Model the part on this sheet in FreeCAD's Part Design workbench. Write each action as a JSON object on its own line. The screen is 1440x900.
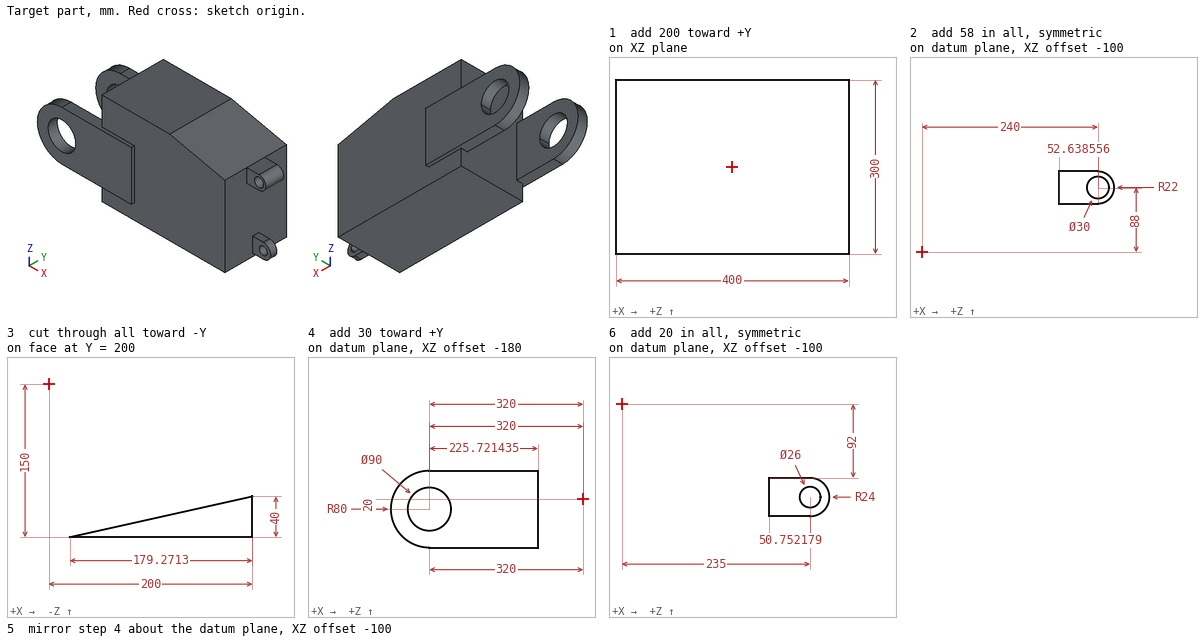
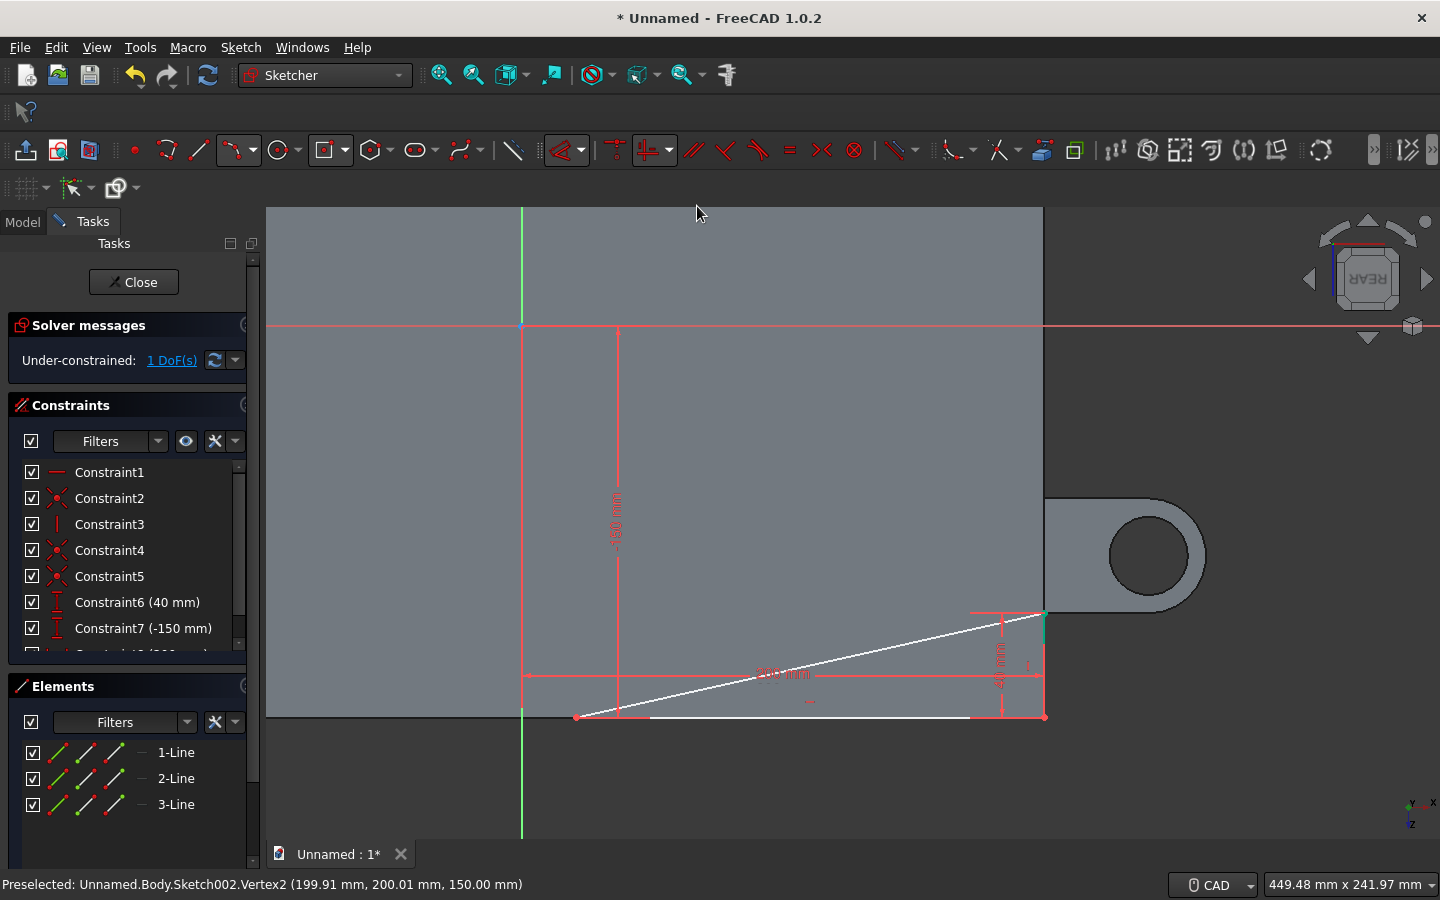
{"action": "left_click", "coordinate": [716, 718]}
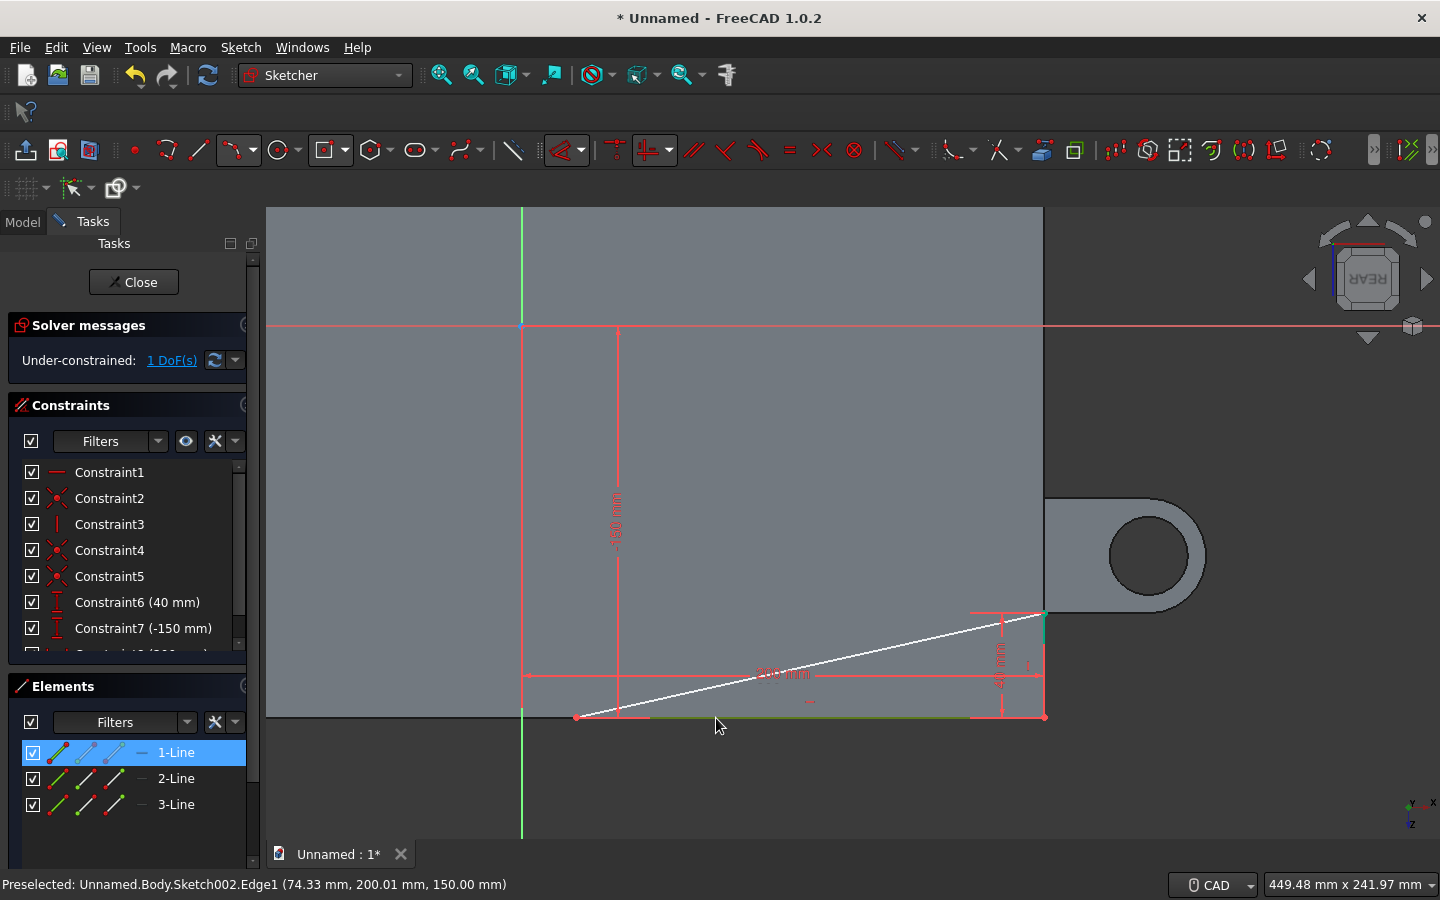
{"action": "key", "text": "l"}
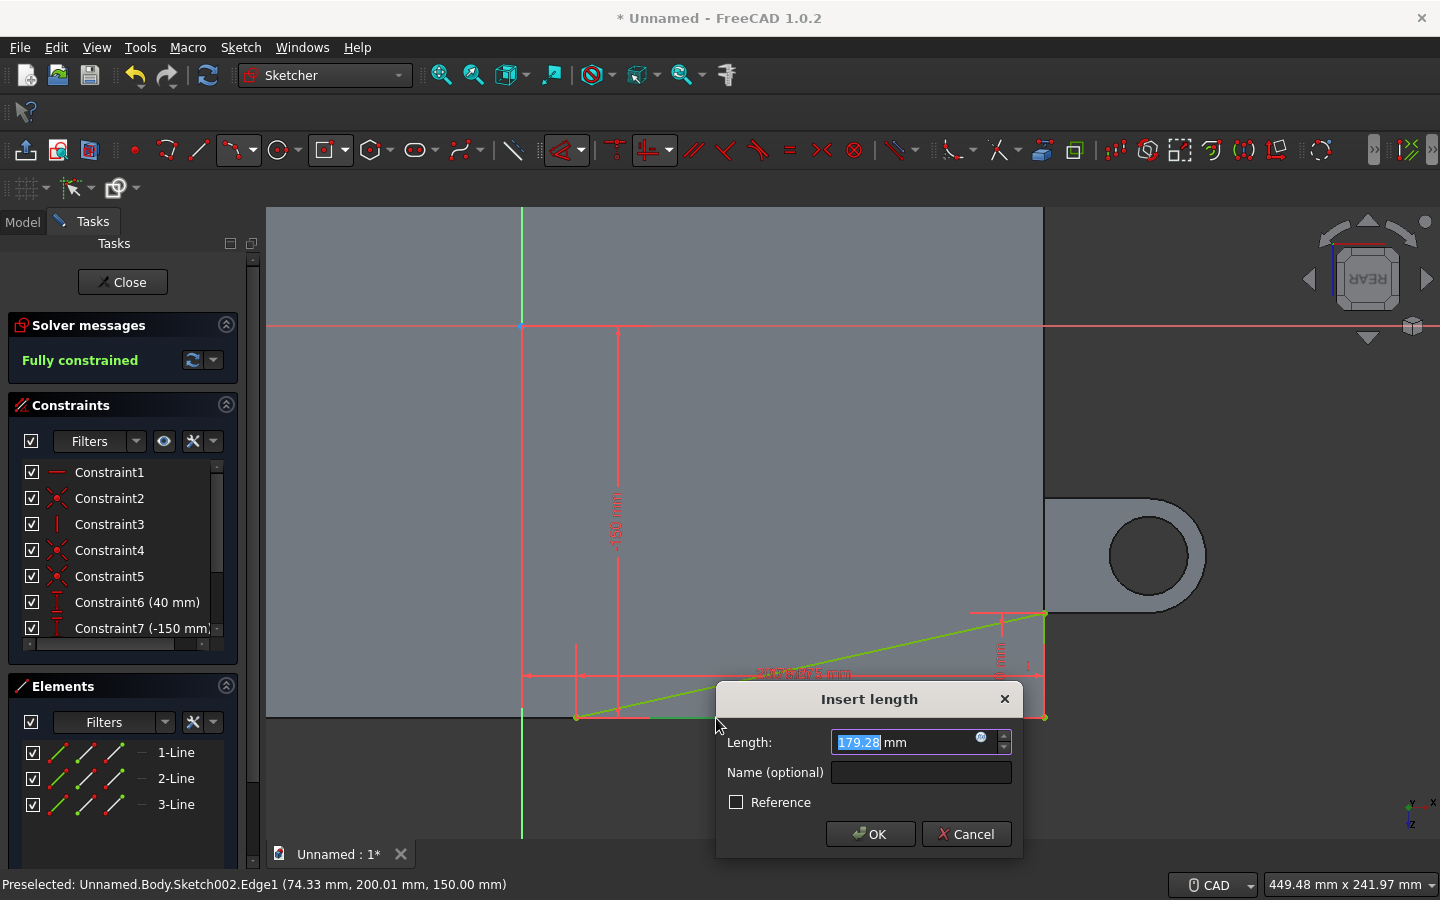
{"action": "type", "text": "179.2713"}
{"action": "key", "text": "Return"}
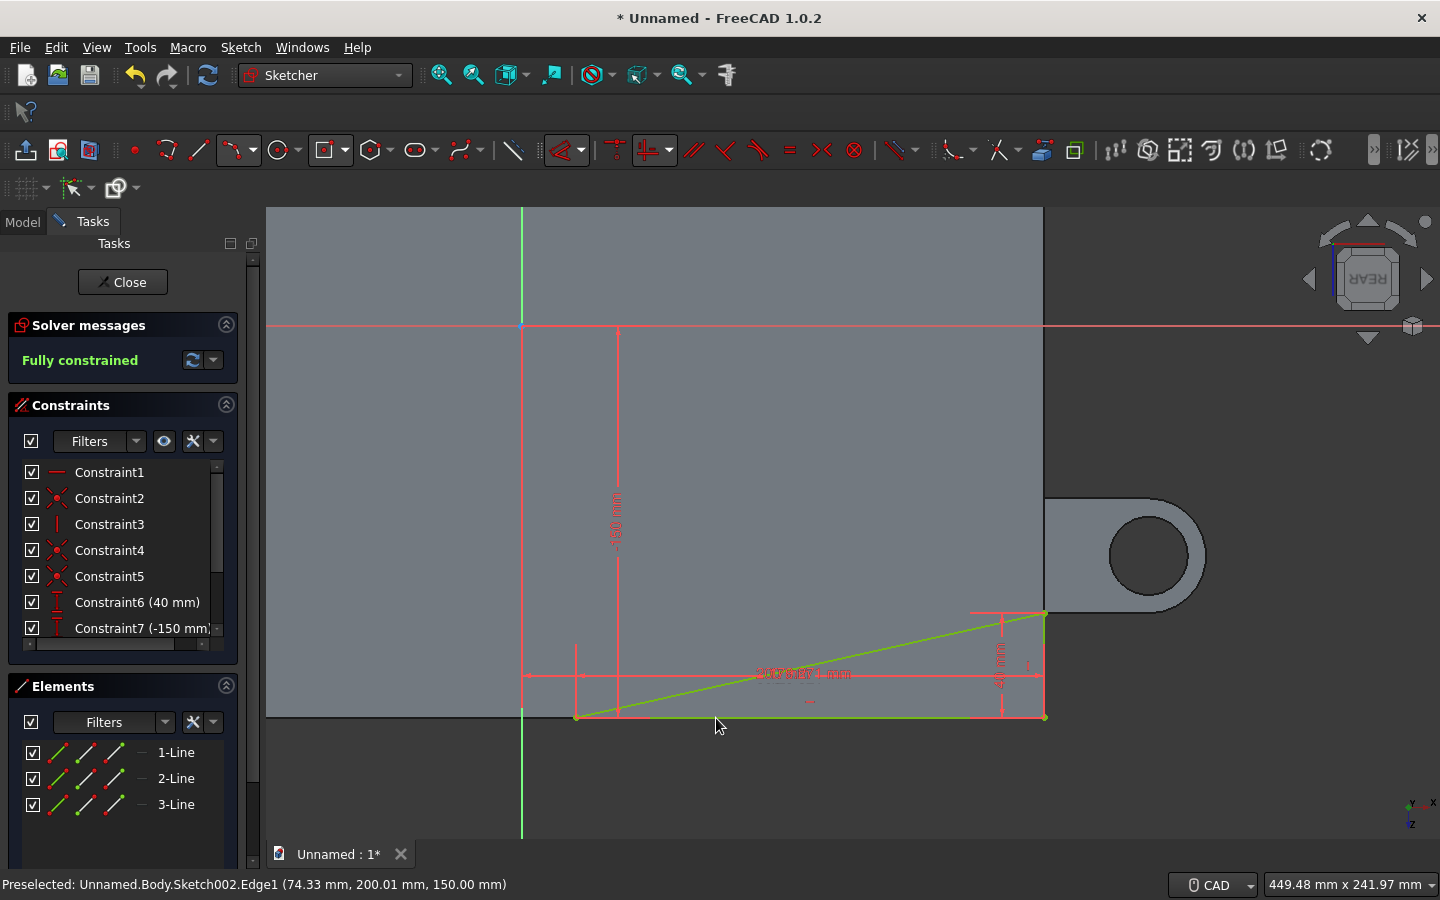
{"action": "left_click", "coordinate": [123, 282]}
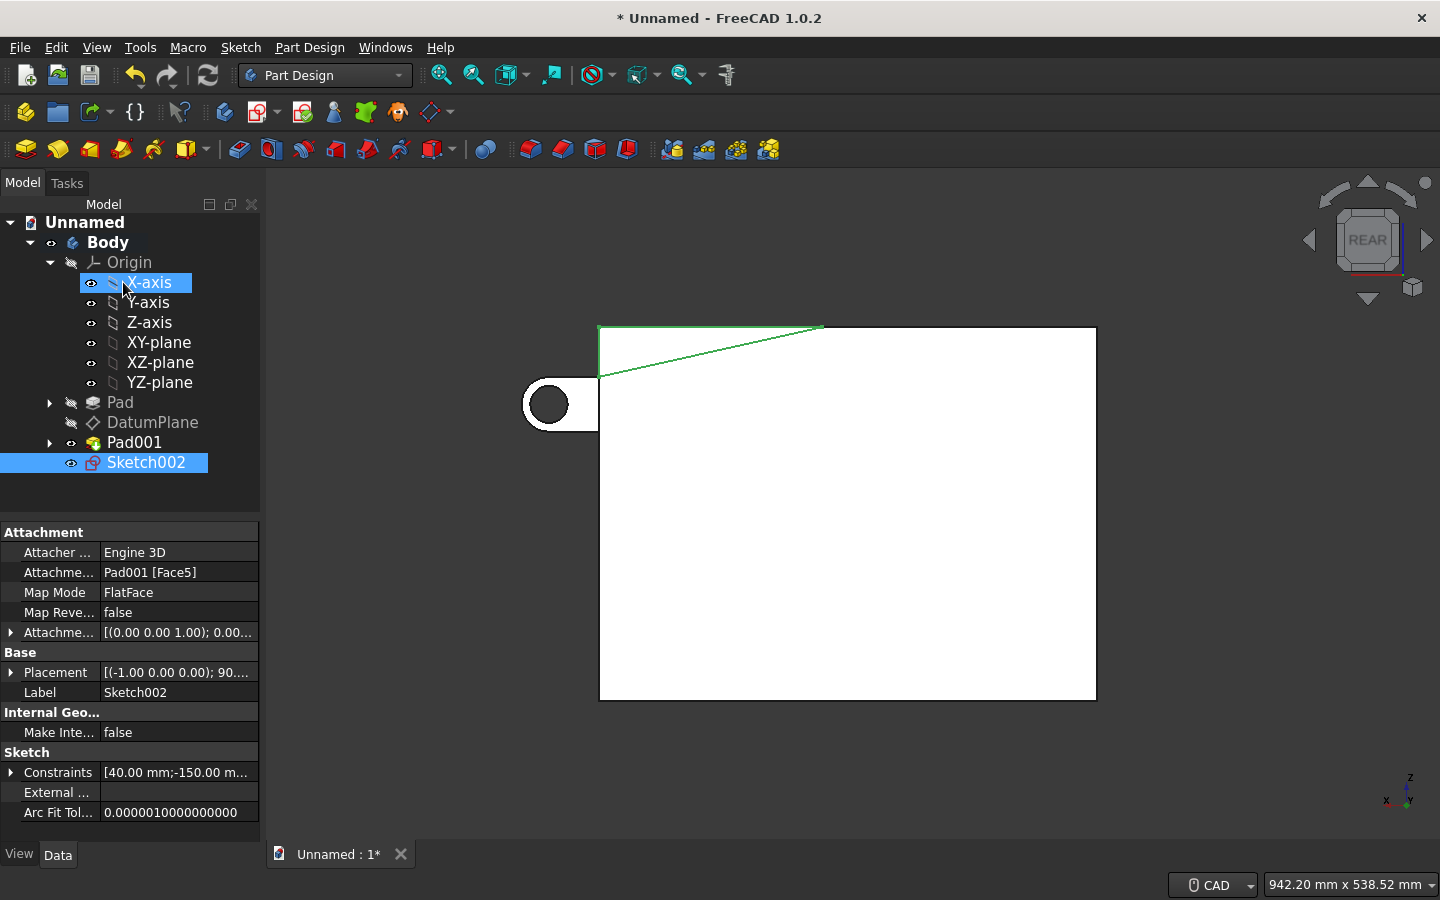
{"action": "left_click", "coordinate": [240, 150]}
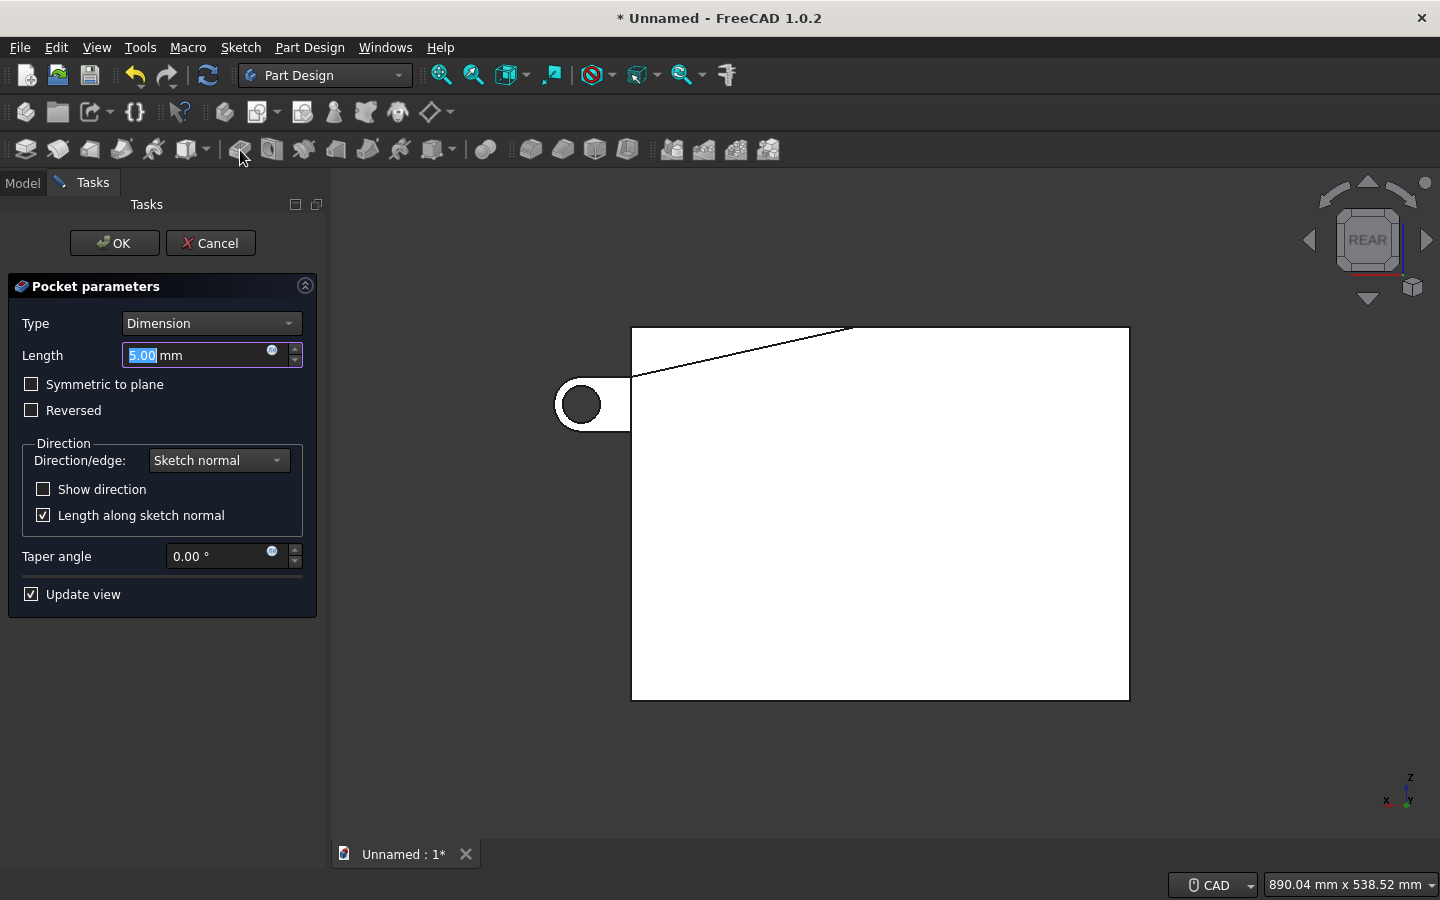
{"action": "left_click", "coordinate": [212, 324]}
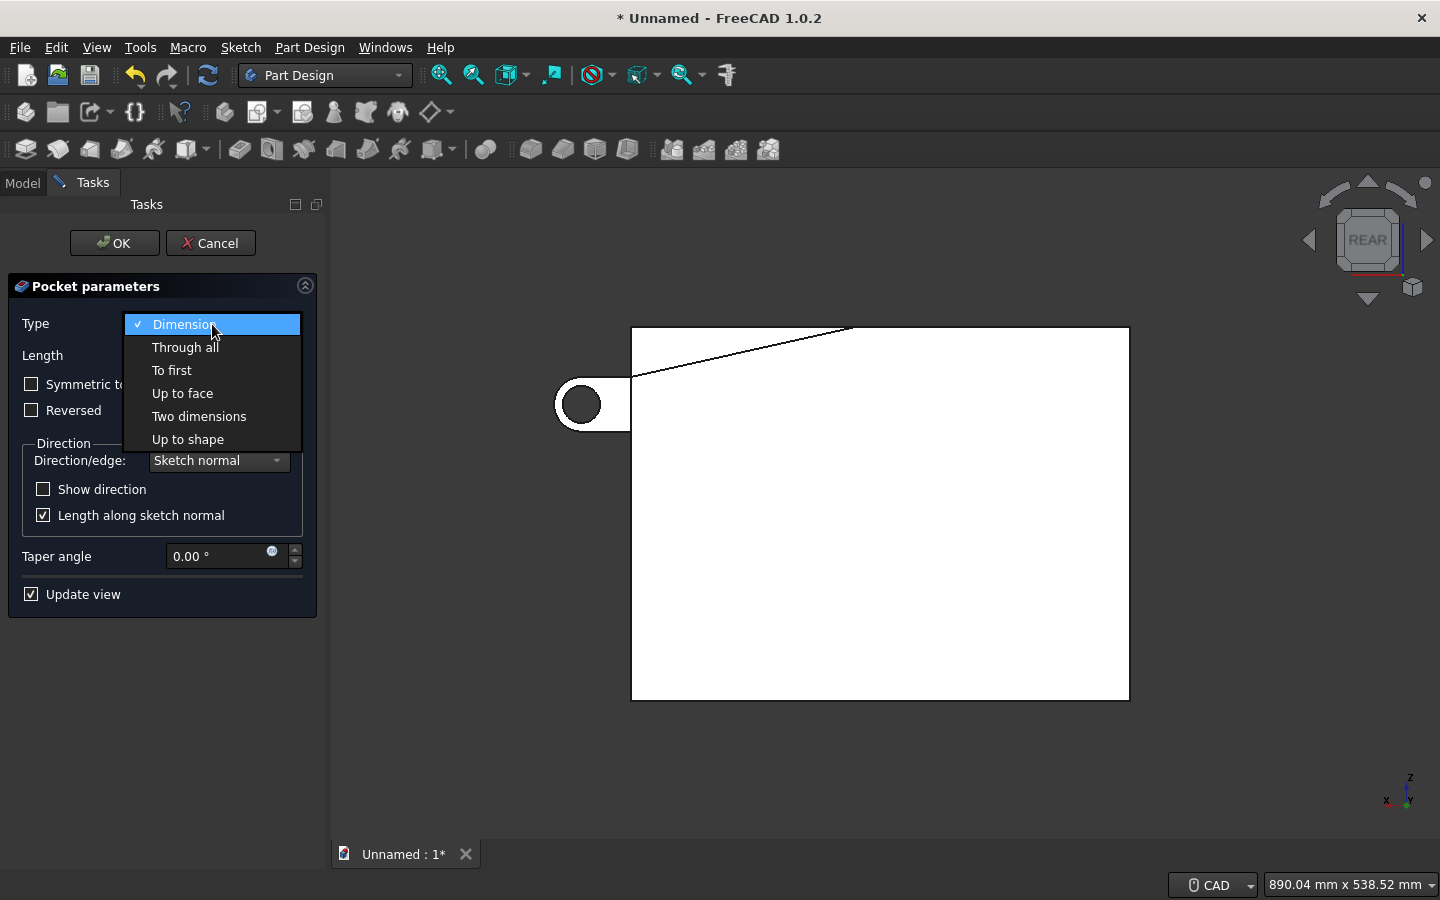
{"action": "left_click", "coordinate": [212, 348]}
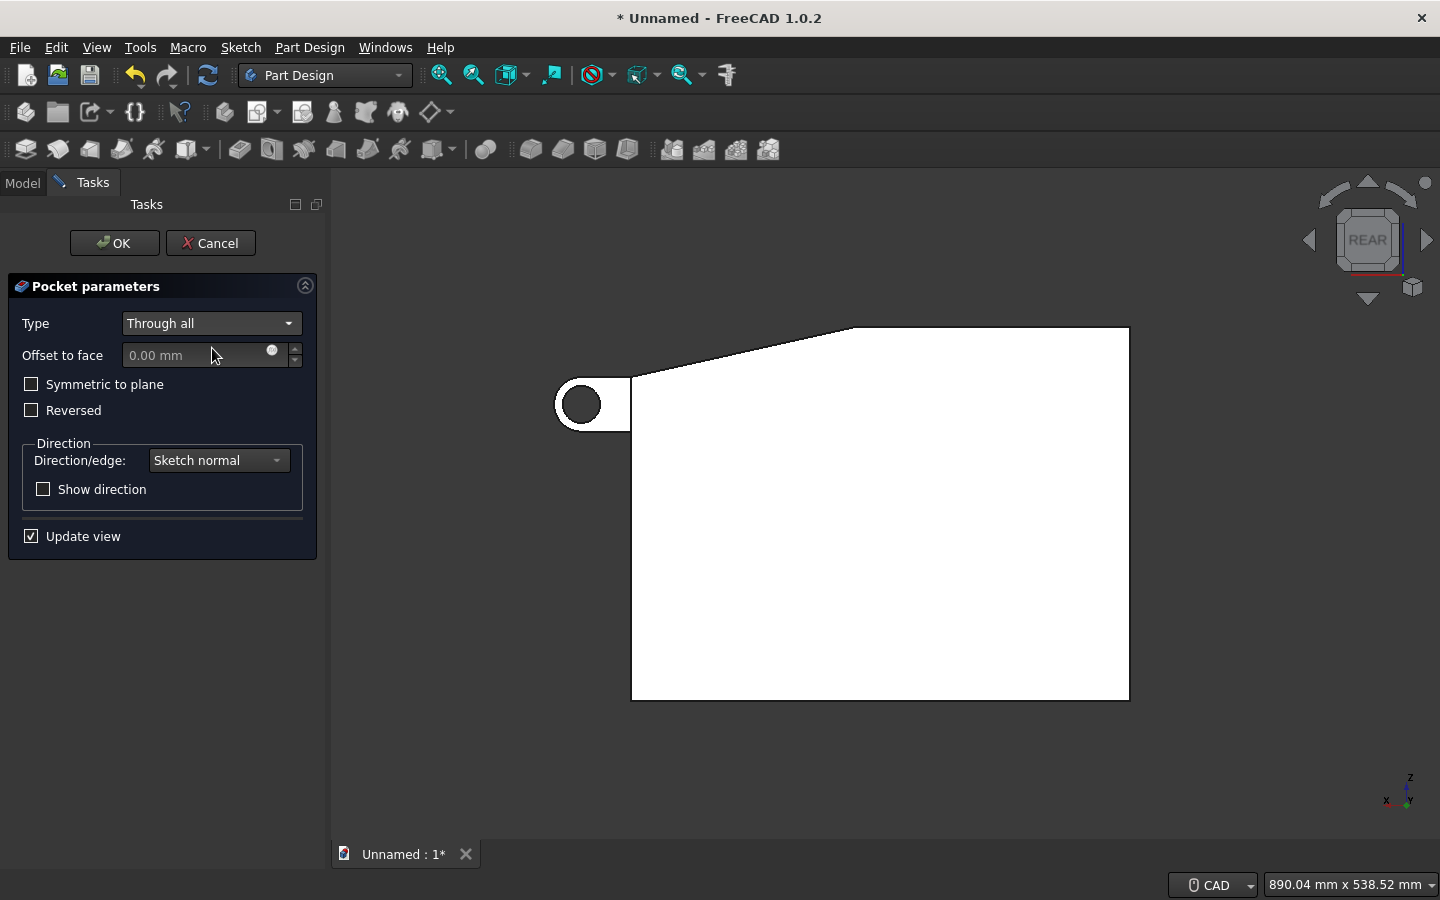
{"action": "left_click", "coordinate": [115, 243]}